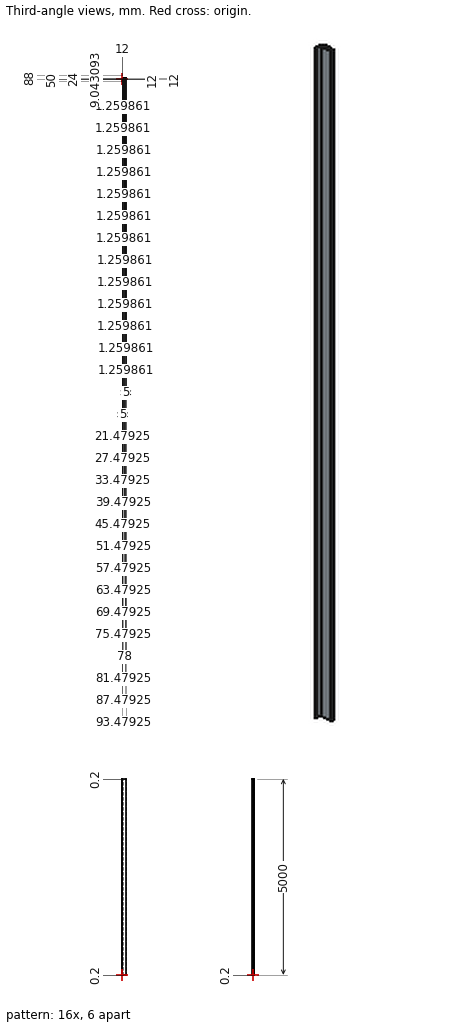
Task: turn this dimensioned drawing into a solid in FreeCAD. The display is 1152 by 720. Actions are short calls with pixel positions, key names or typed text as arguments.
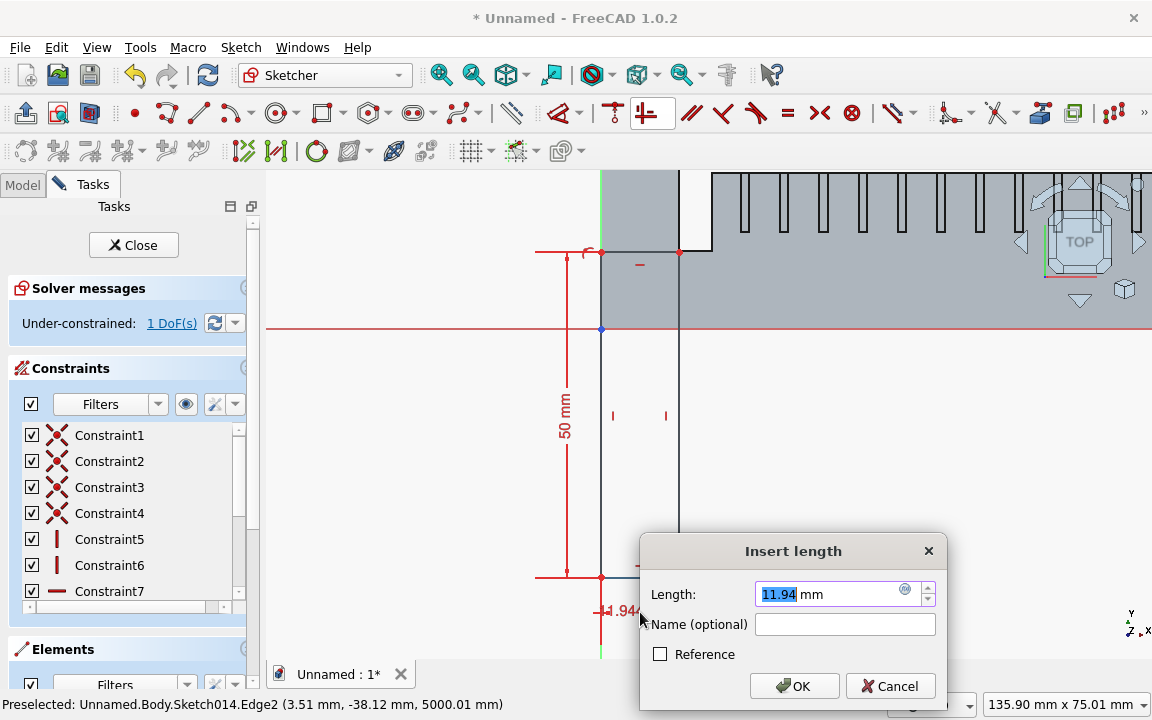
text(12)
key(Return)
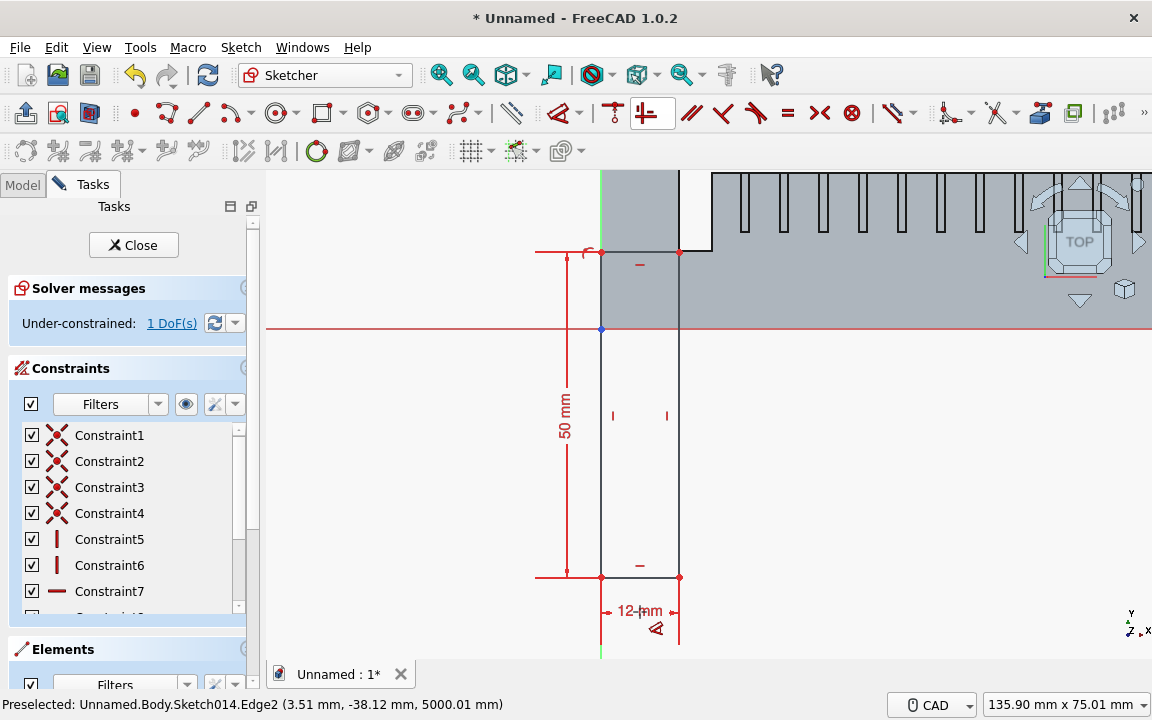
click(601, 252)
click(567, 291)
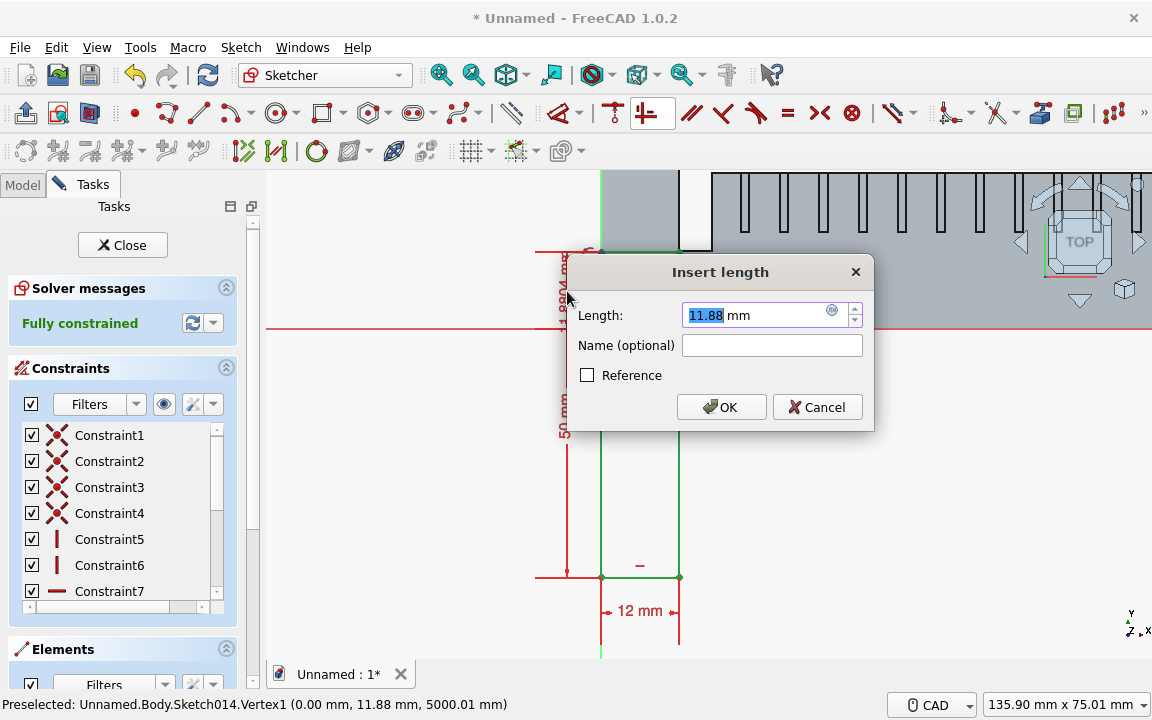
text(12)
key(Return)
key(Escape)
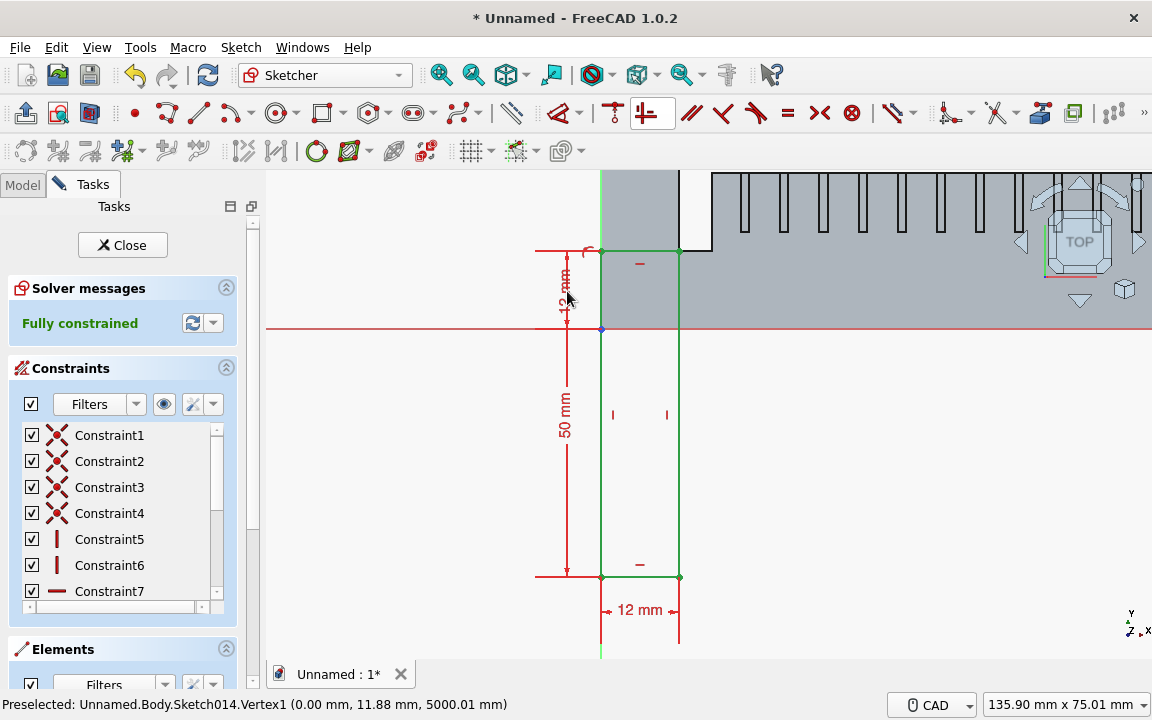
click(123, 245)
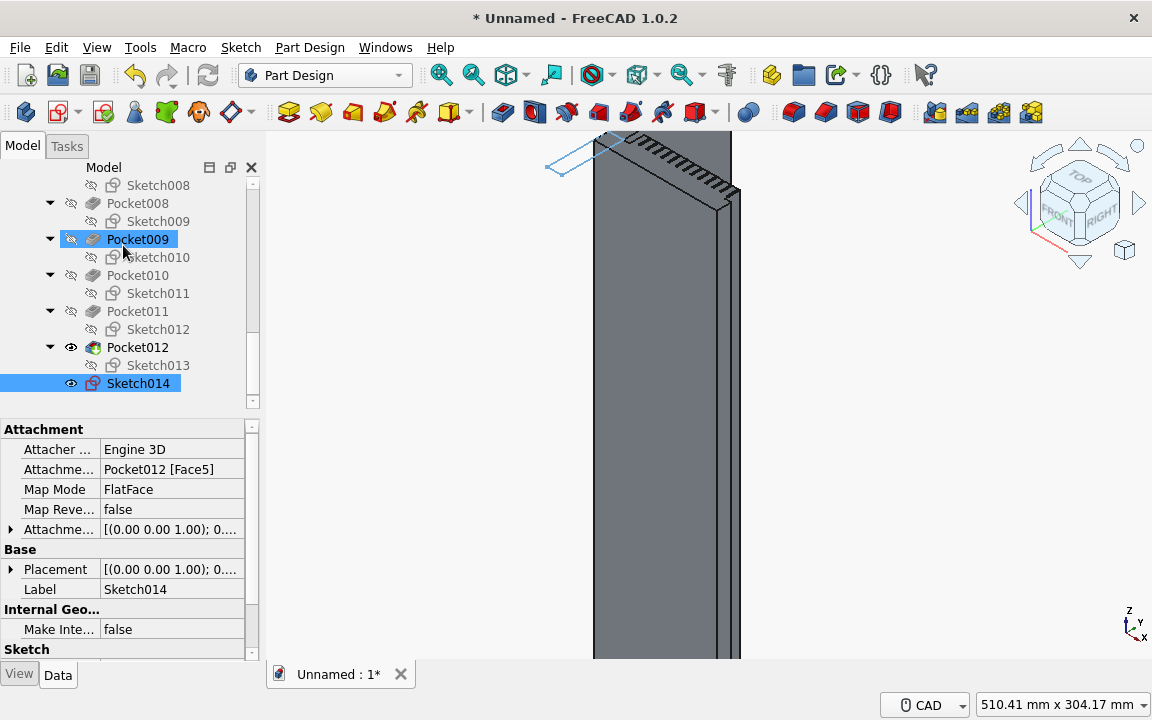
click(290, 112)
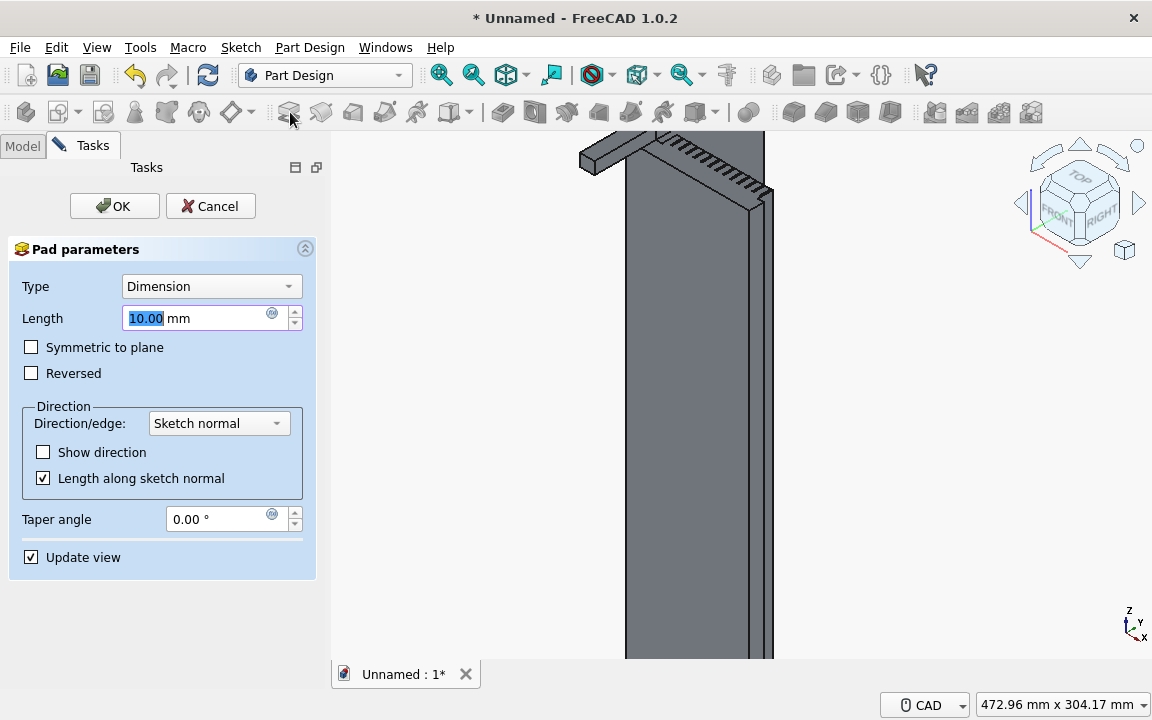
text(5000)
key(Tab)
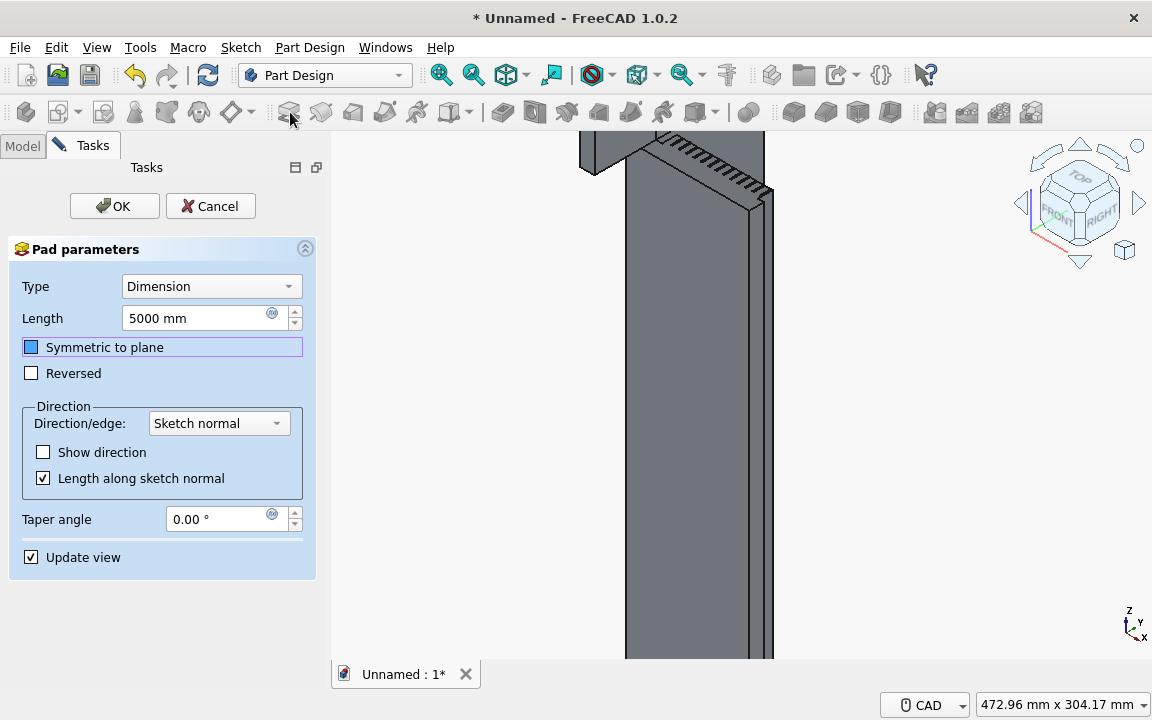
click(30, 373)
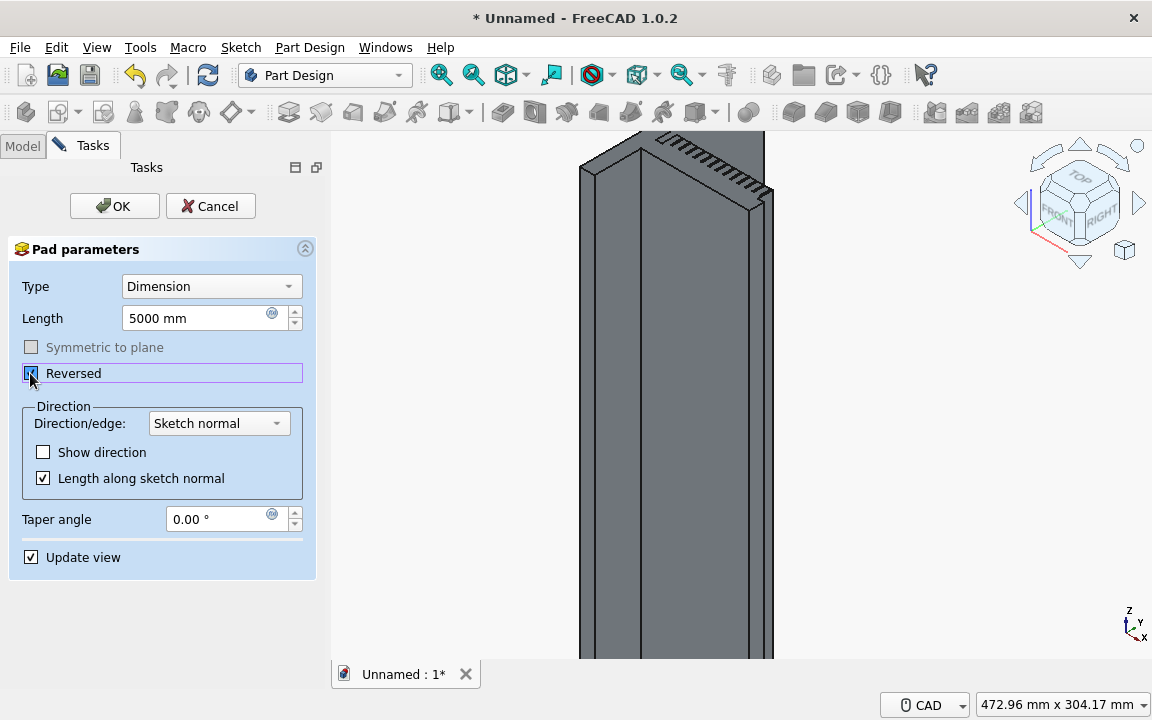
click(115, 206)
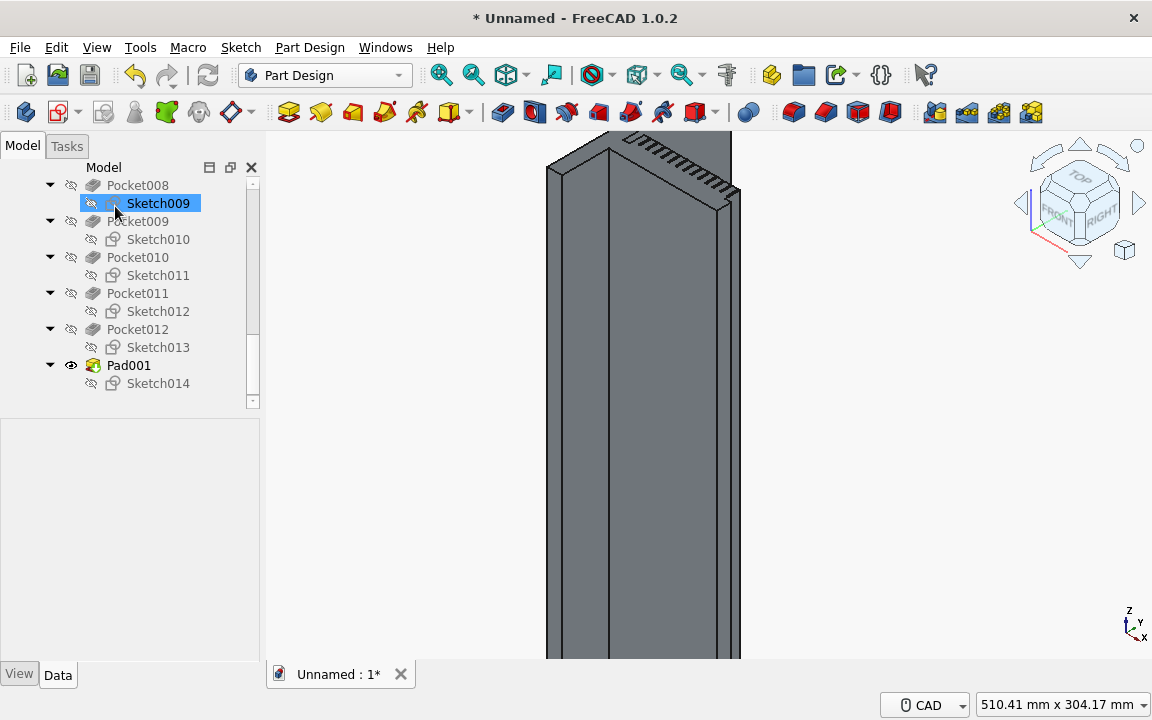
click(442, 76)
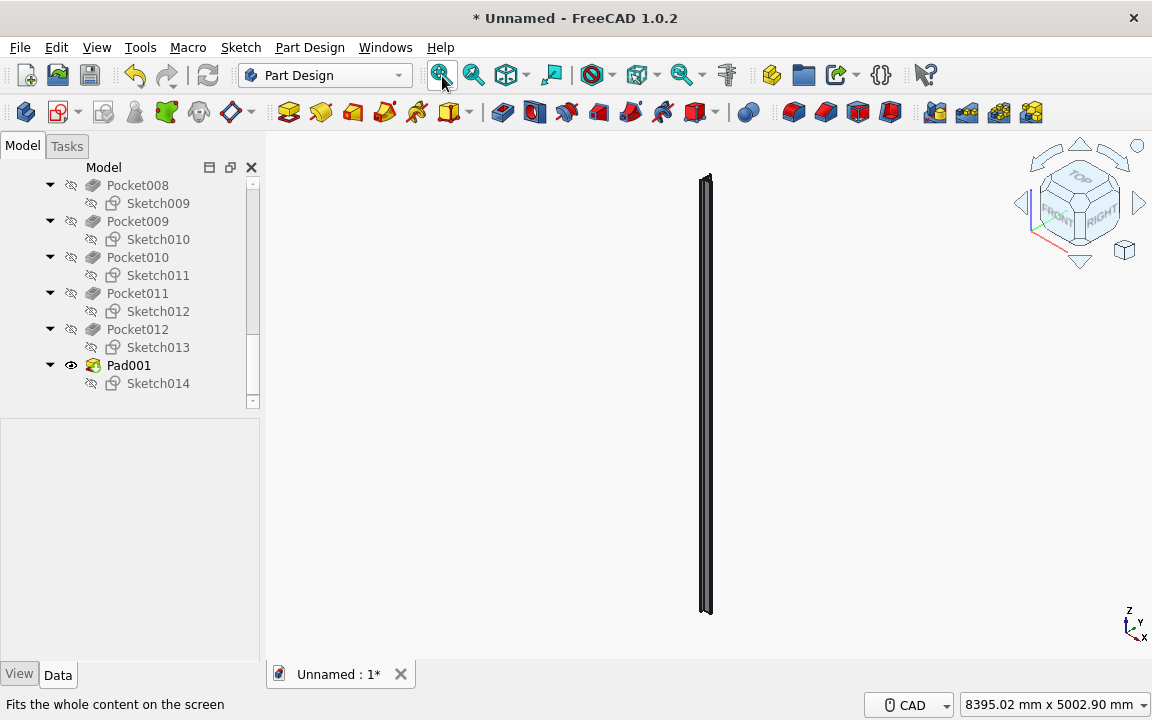
click(58, 112)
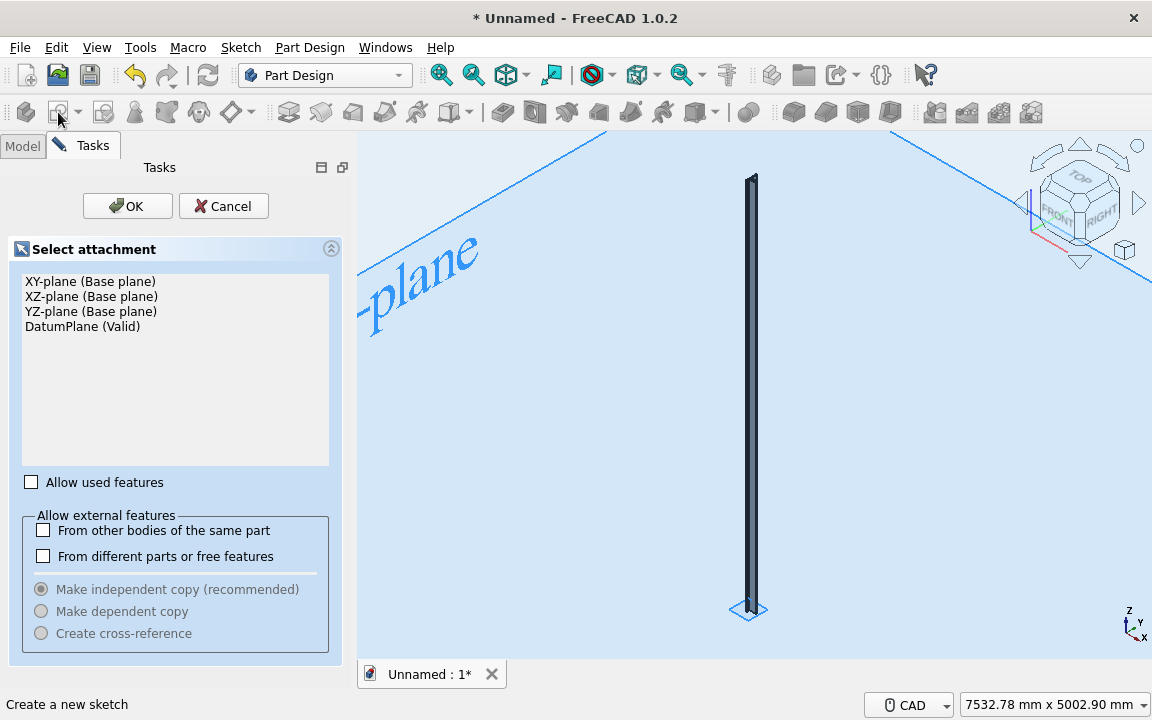
click(82, 282)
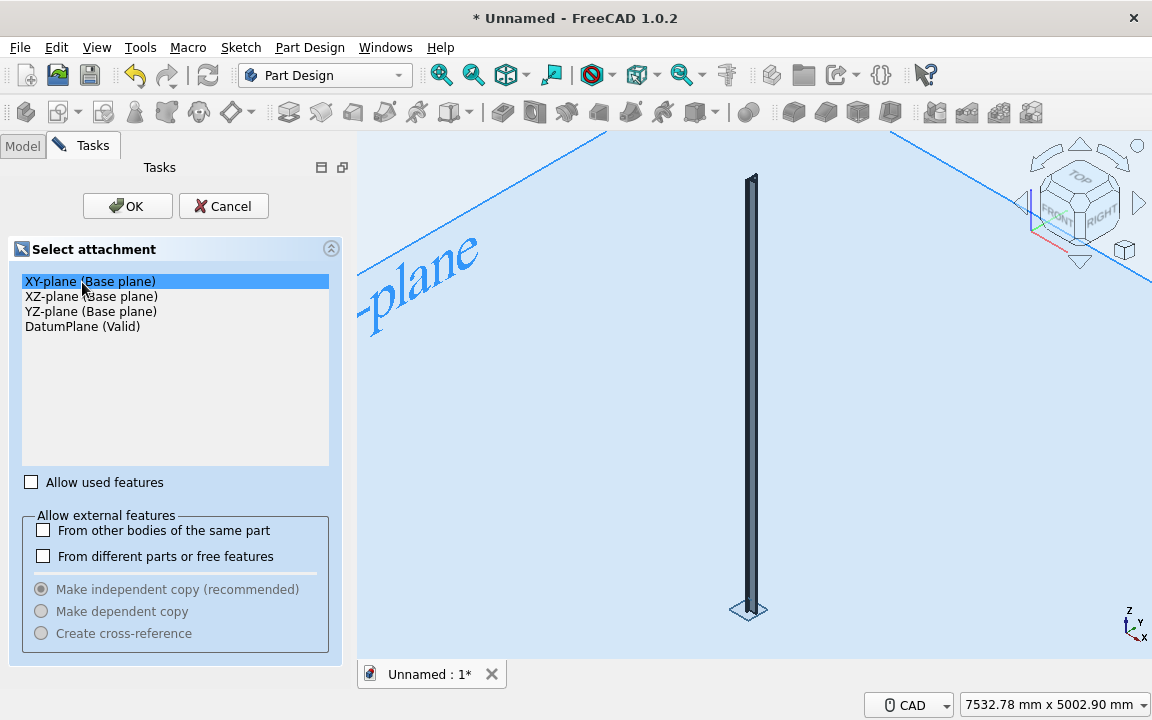
click(128, 206)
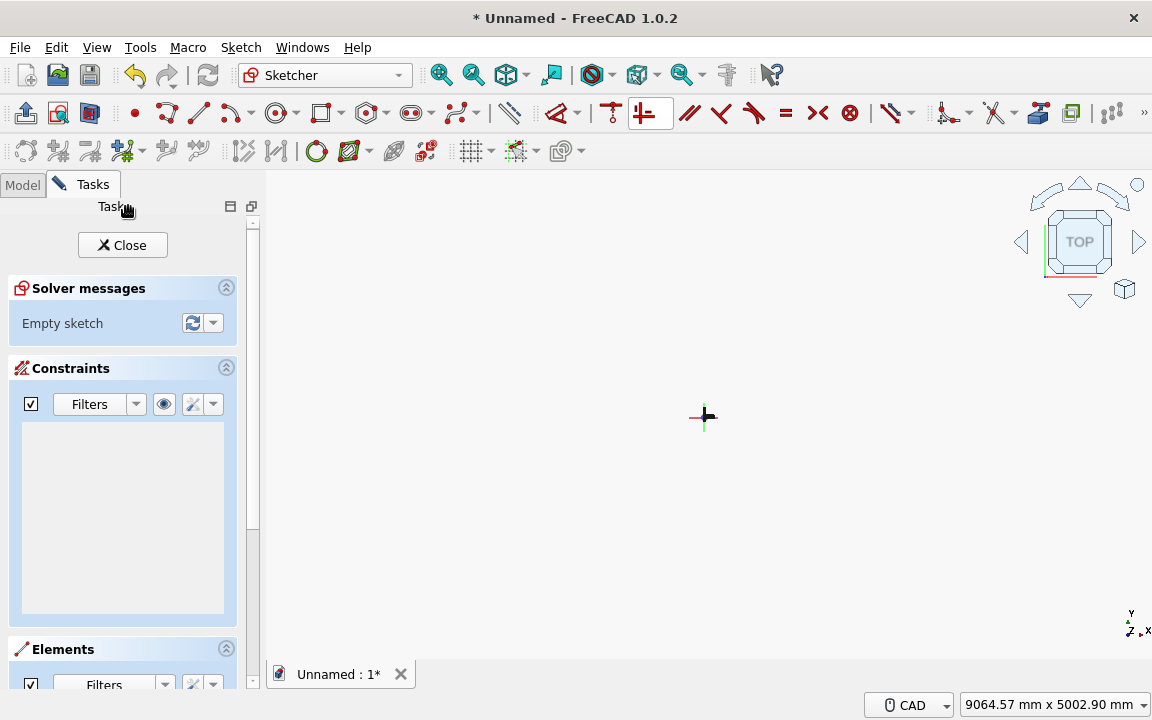
click(90, 114)